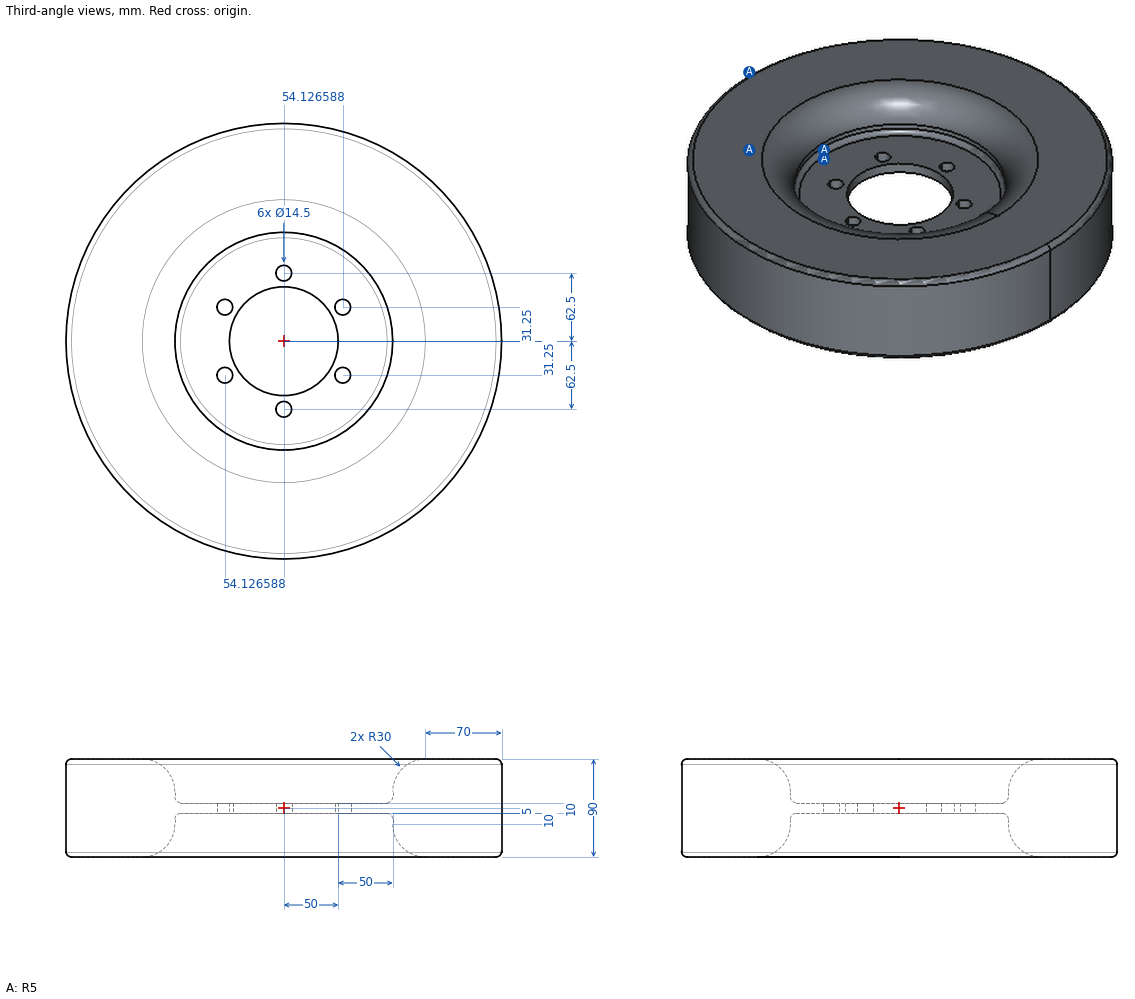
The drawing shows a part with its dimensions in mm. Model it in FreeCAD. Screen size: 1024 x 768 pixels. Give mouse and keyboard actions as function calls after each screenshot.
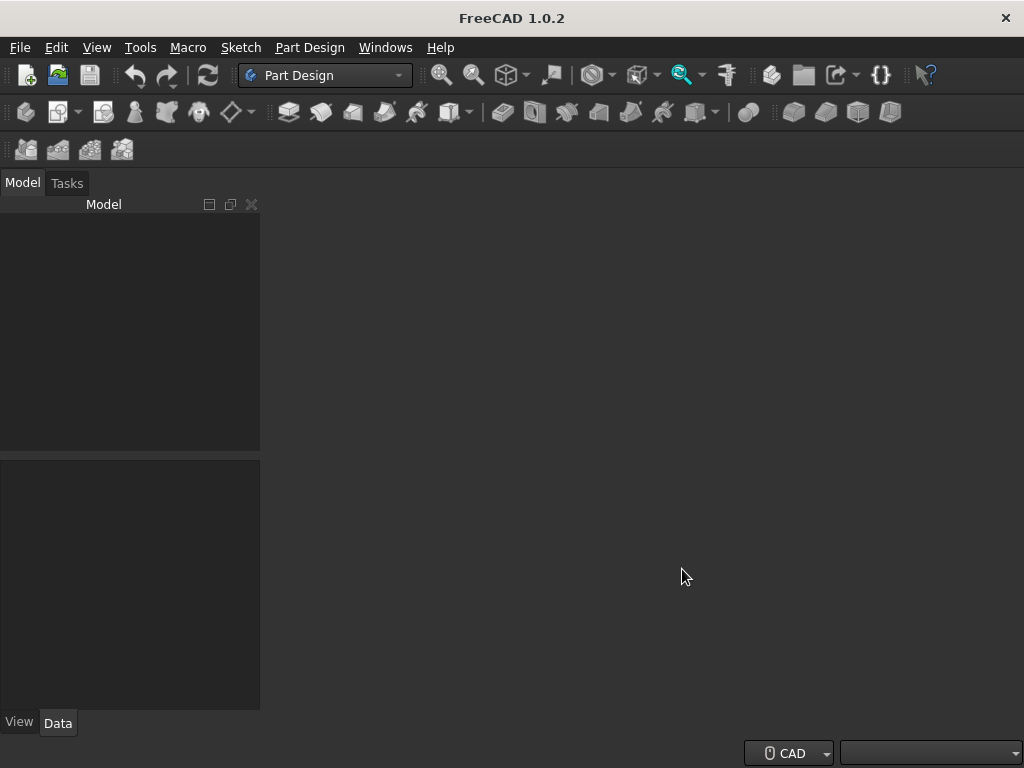
click(26, 76)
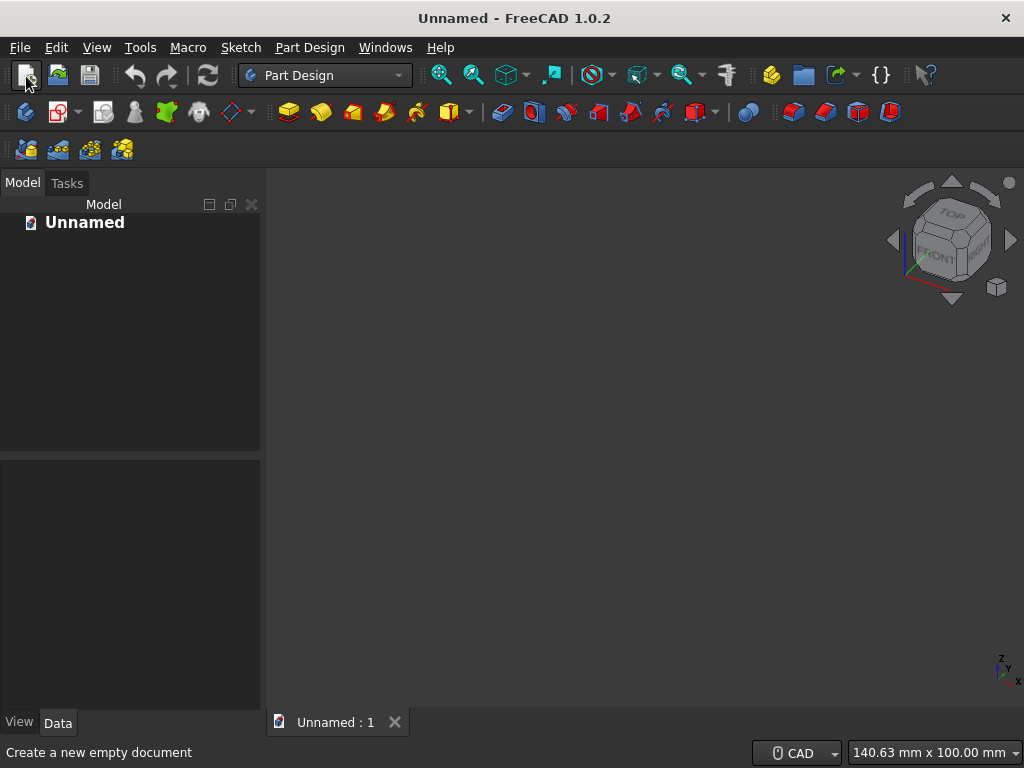
click(58, 112)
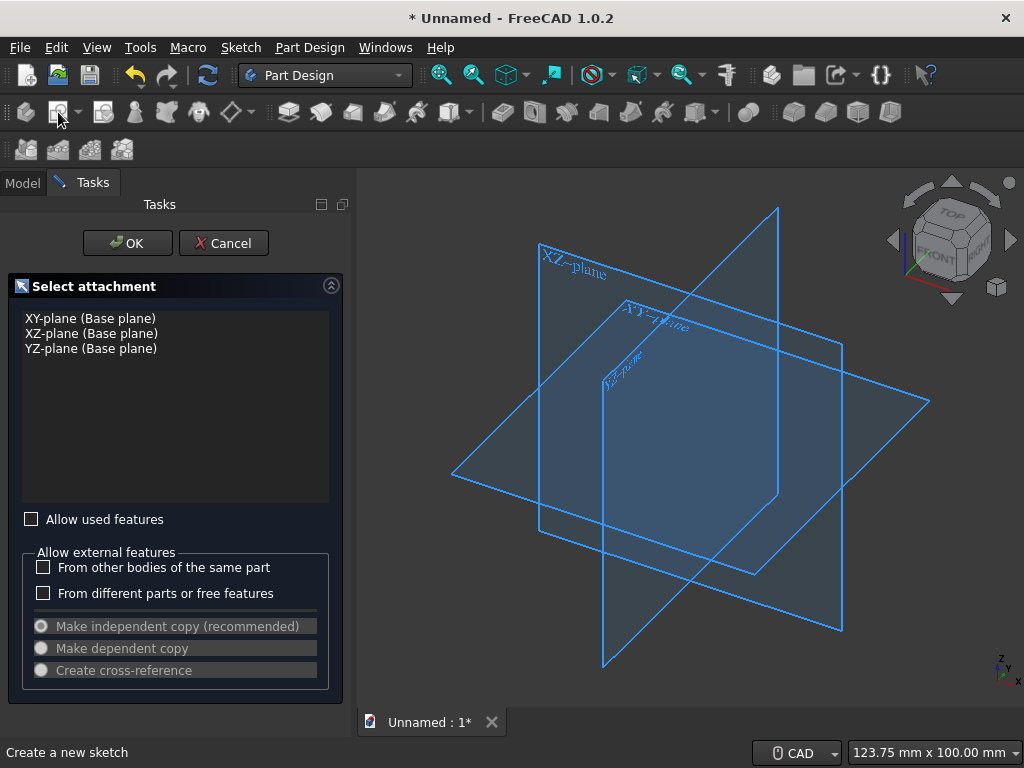
click(82, 334)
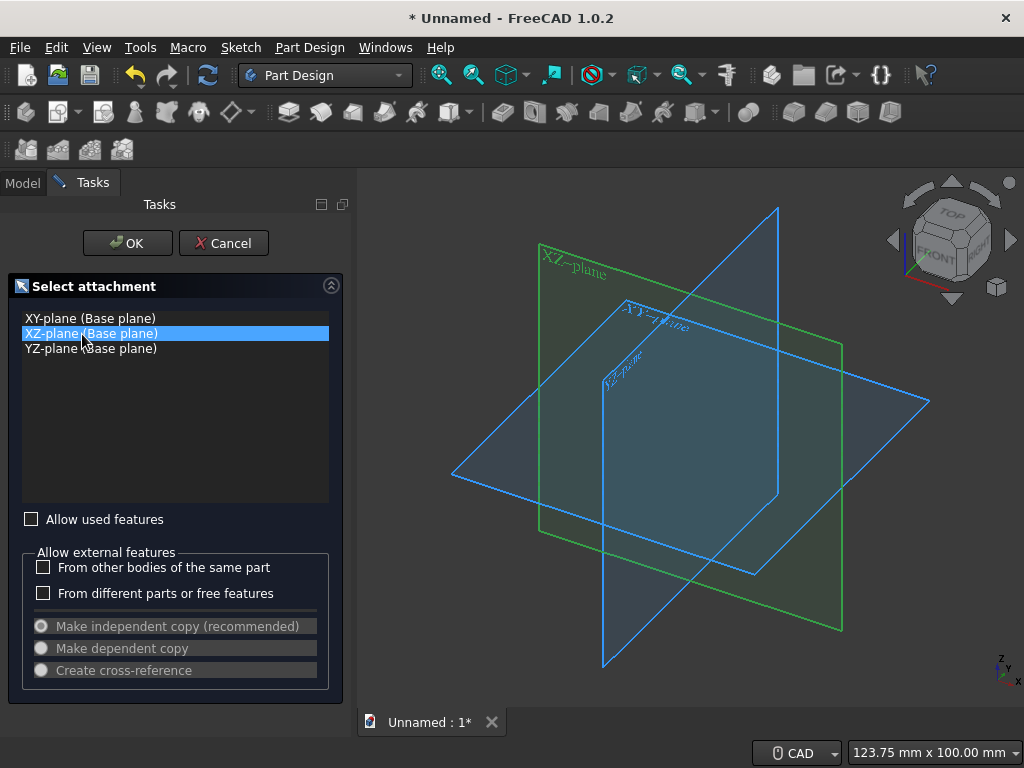
click(128, 243)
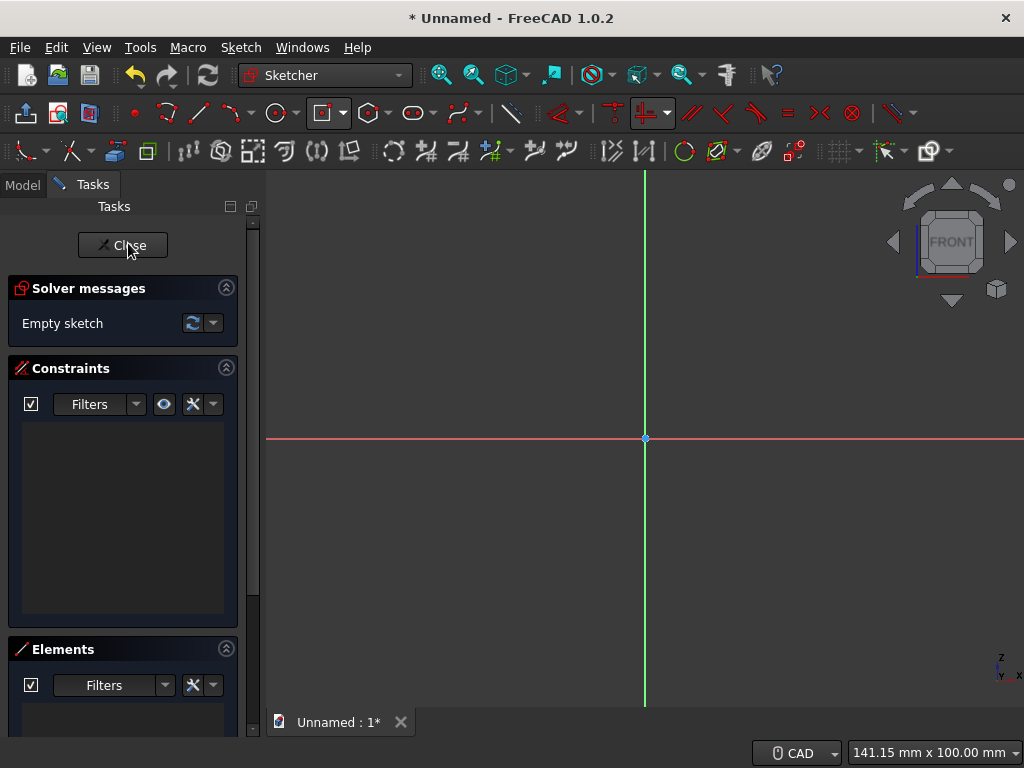
scroll(294, 439, down, 5)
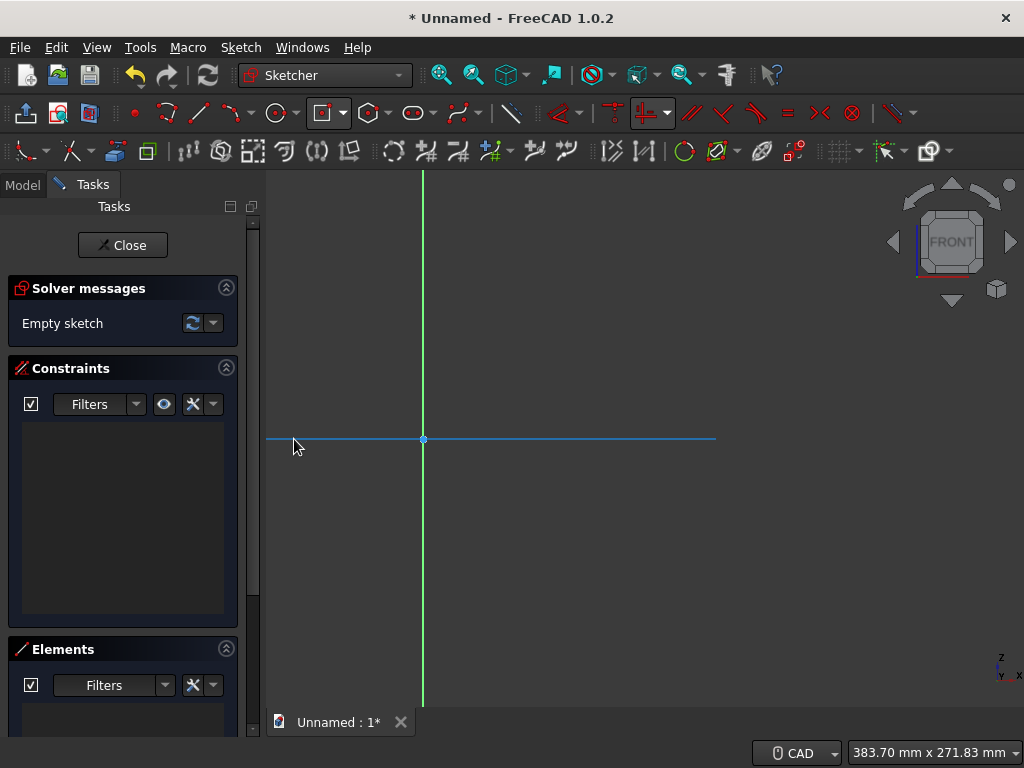
click(168, 114)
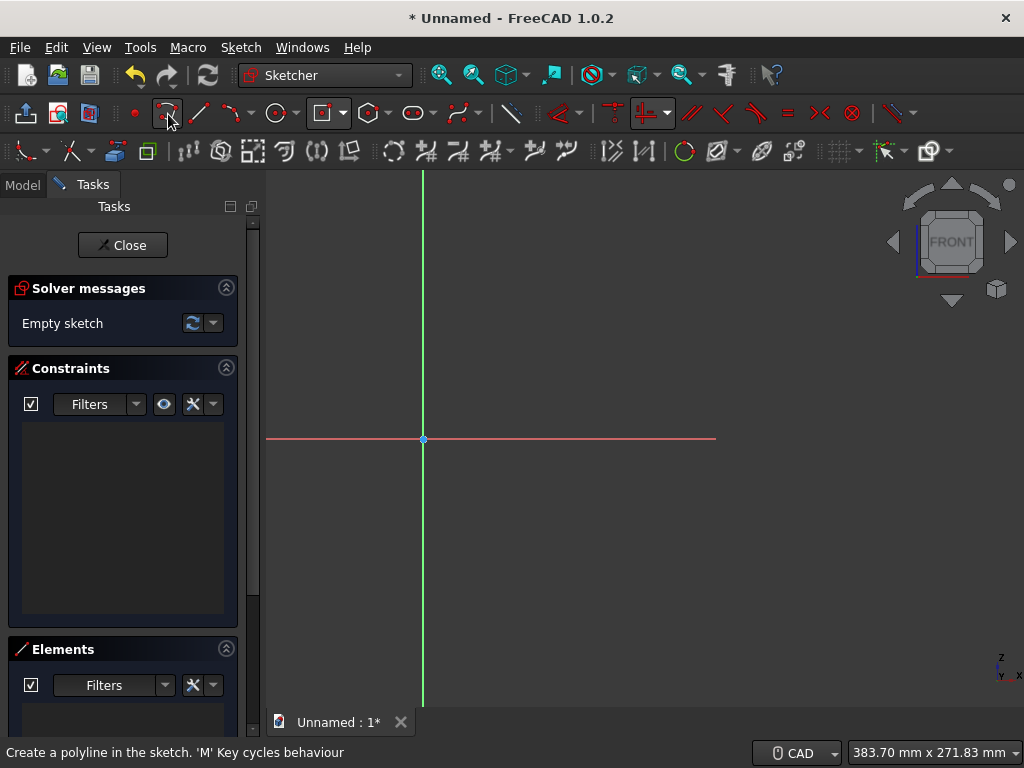
click(680, 350)
click(818, 350)
click(818, 528)
click(680, 528)
right_click(680, 528)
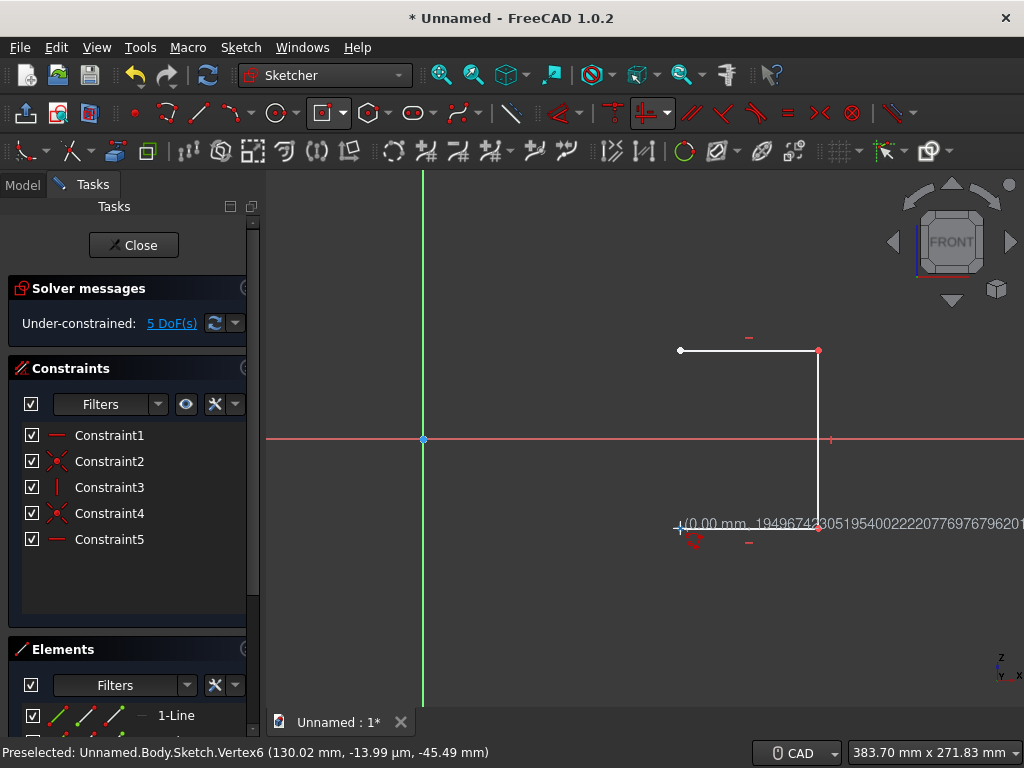
click(621, 469)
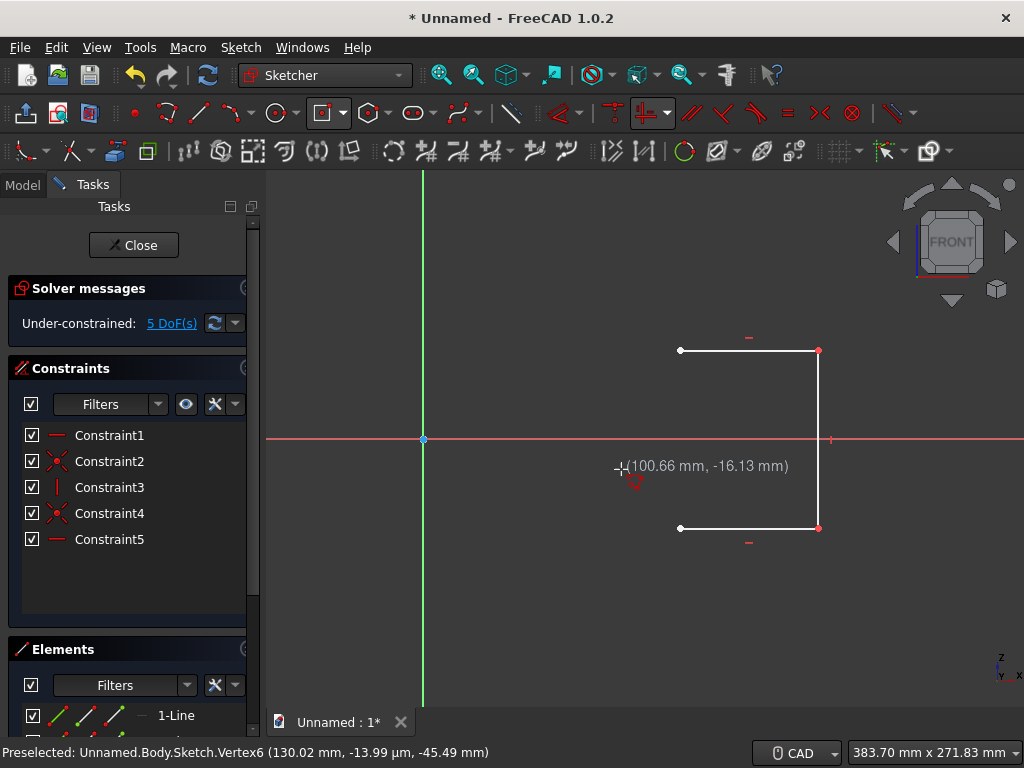
scroll(621, 449, up, 3)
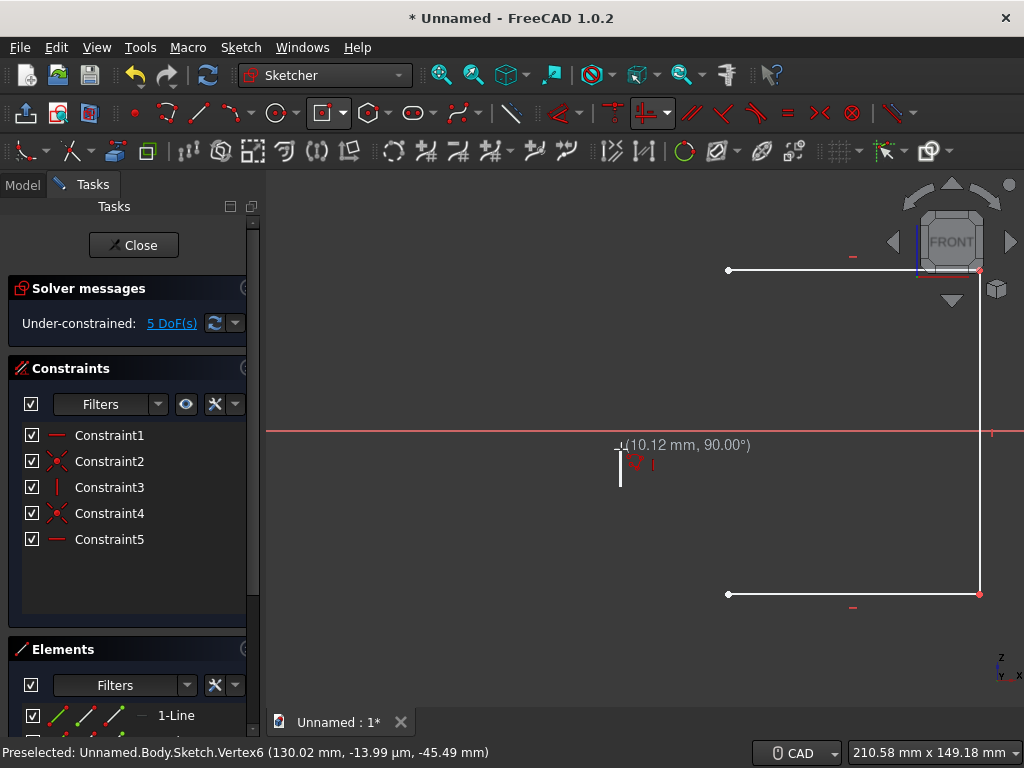
click(621, 449)
click(440, 449)
click(440, 413)
click(620, 413)
click(620, 377)
right_click(620, 377)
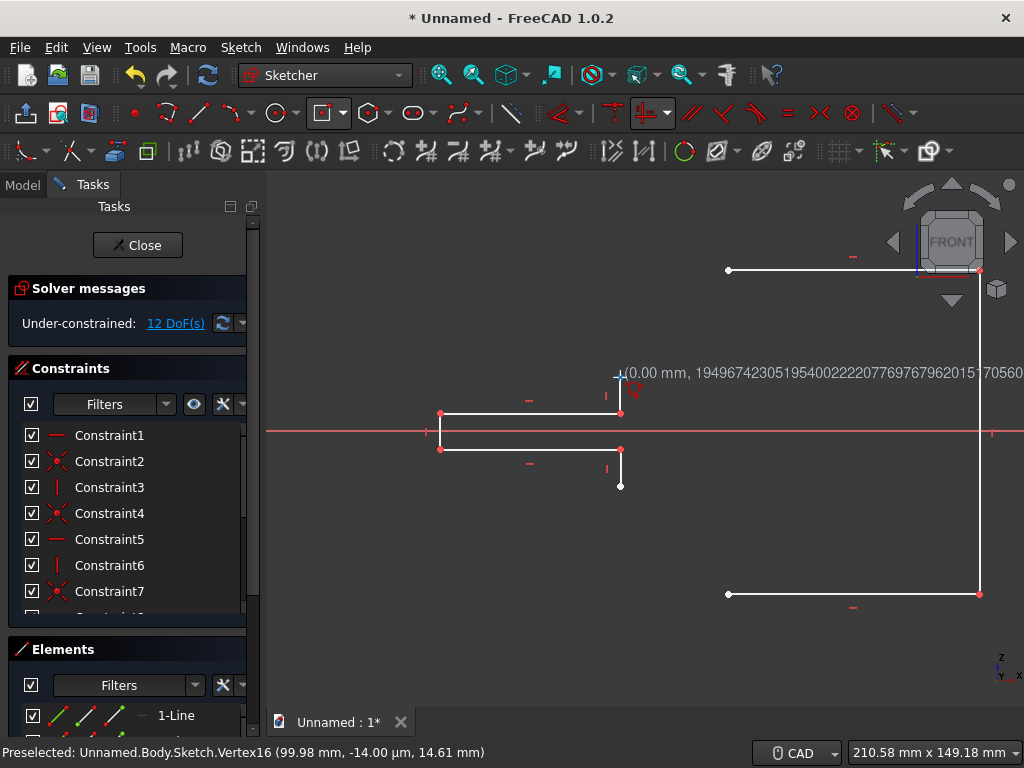
click(232, 114)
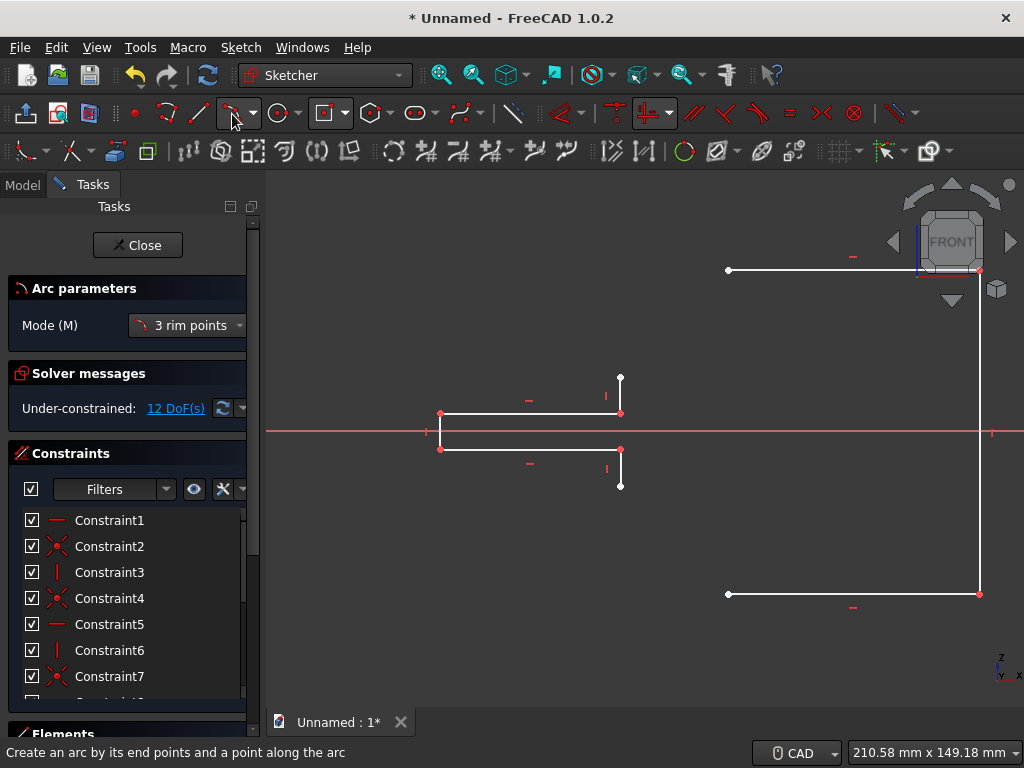
click(728, 594)
click(621, 487)
click(652, 561)